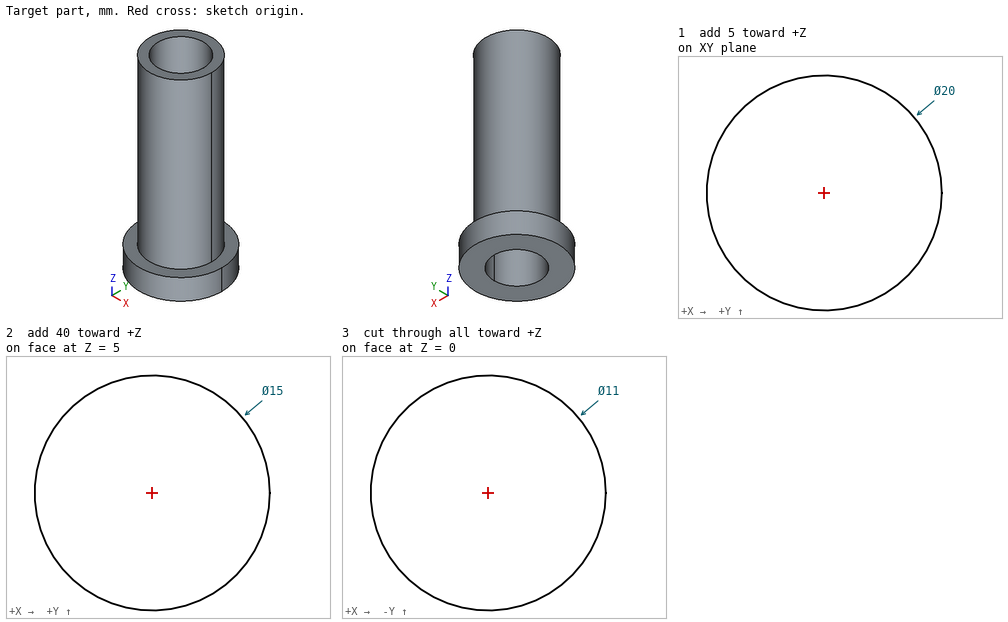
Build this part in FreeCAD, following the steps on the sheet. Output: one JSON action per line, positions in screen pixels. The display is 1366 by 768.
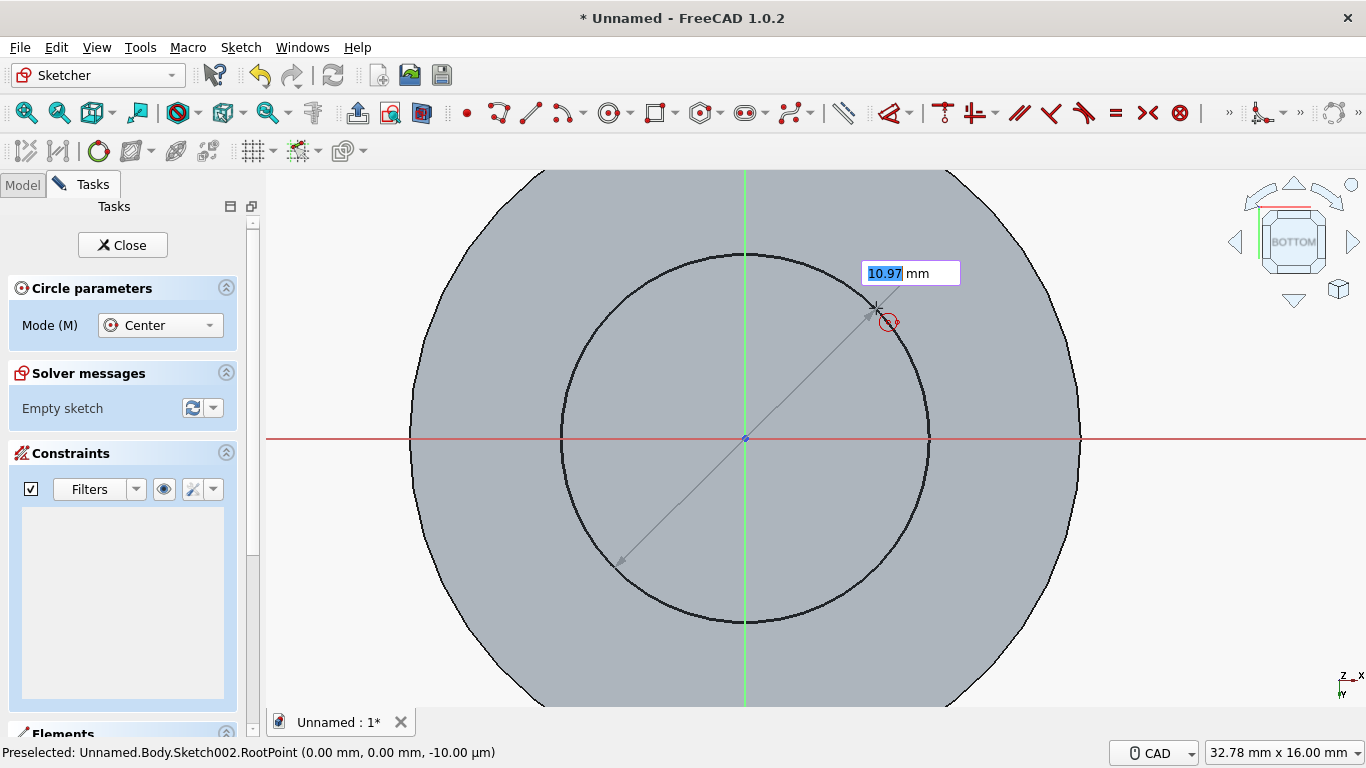
{"action": "type", "text": "11"}
{"action": "key", "text": "Return"}
{"action": "key", "text": "Escape"}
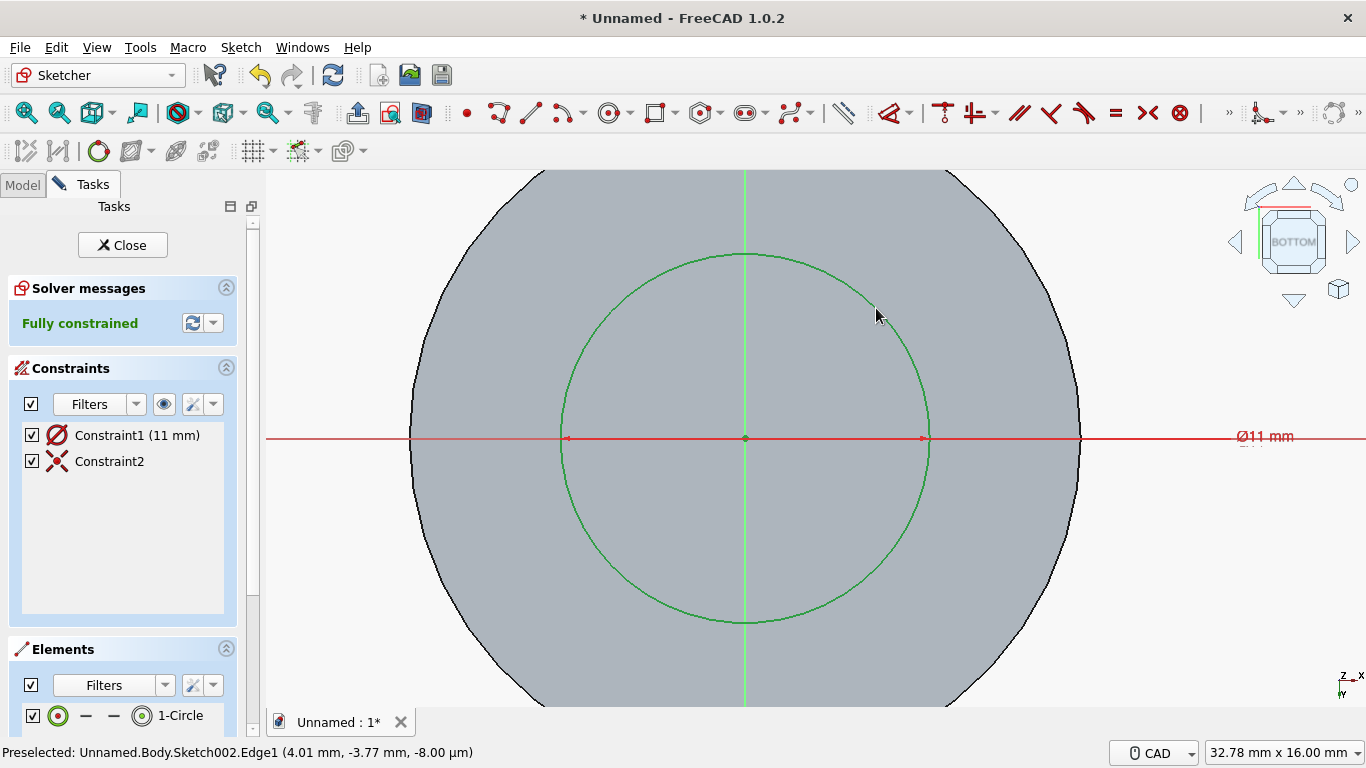
{"action": "left_click", "coordinate": [123, 245]}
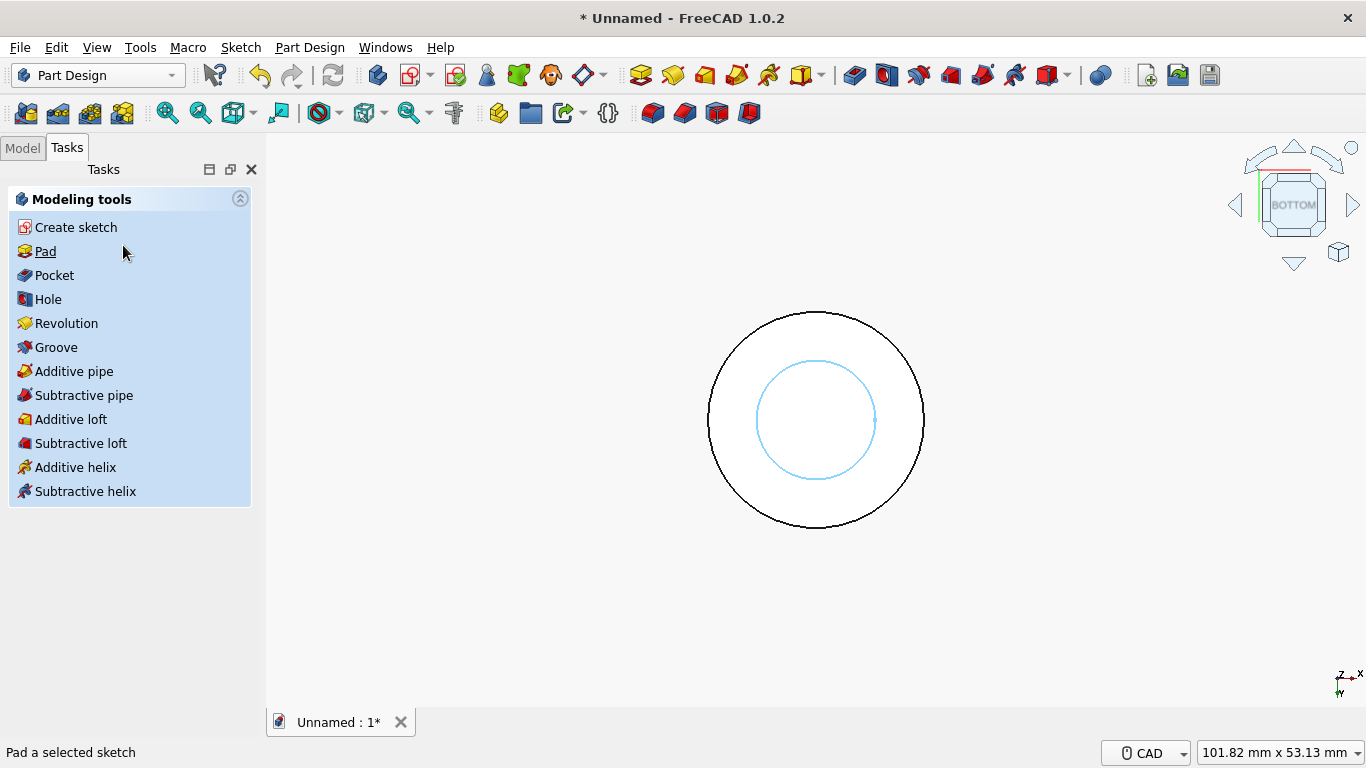
{"action": "left_click", "coordinate": [856, 76]}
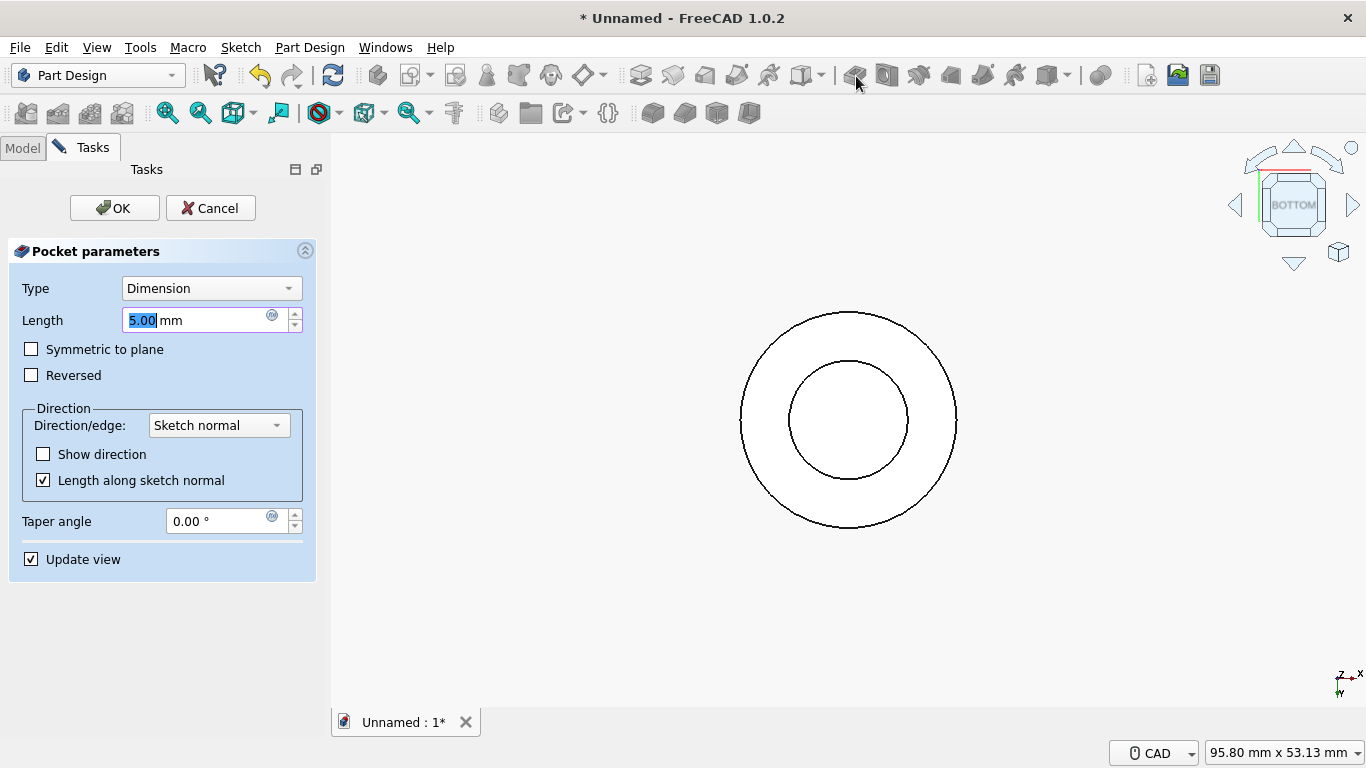
{"action": "left_click", "coordinate": [212, 288]}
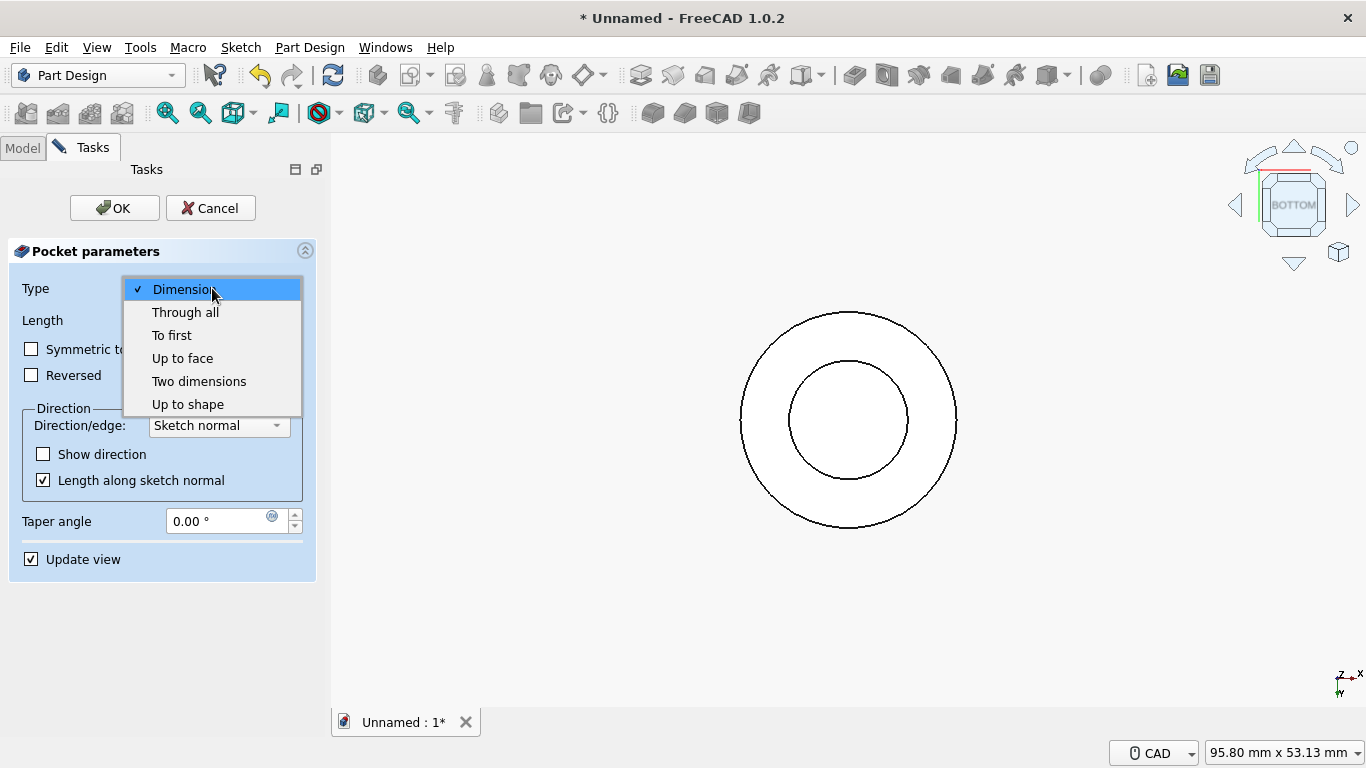
{"action": "left_click", "coordinate": [212, 312]}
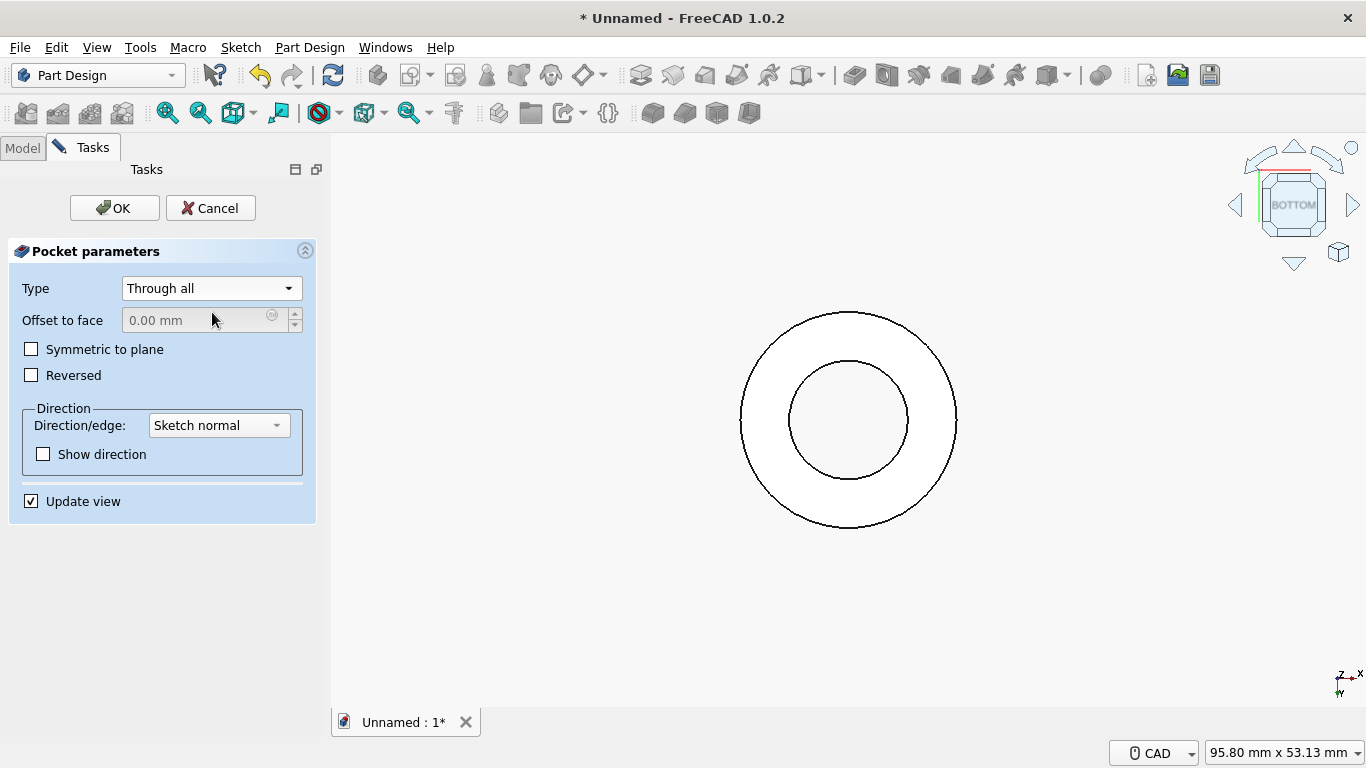
{"action": "left_click", "coordinate": [115, 208]}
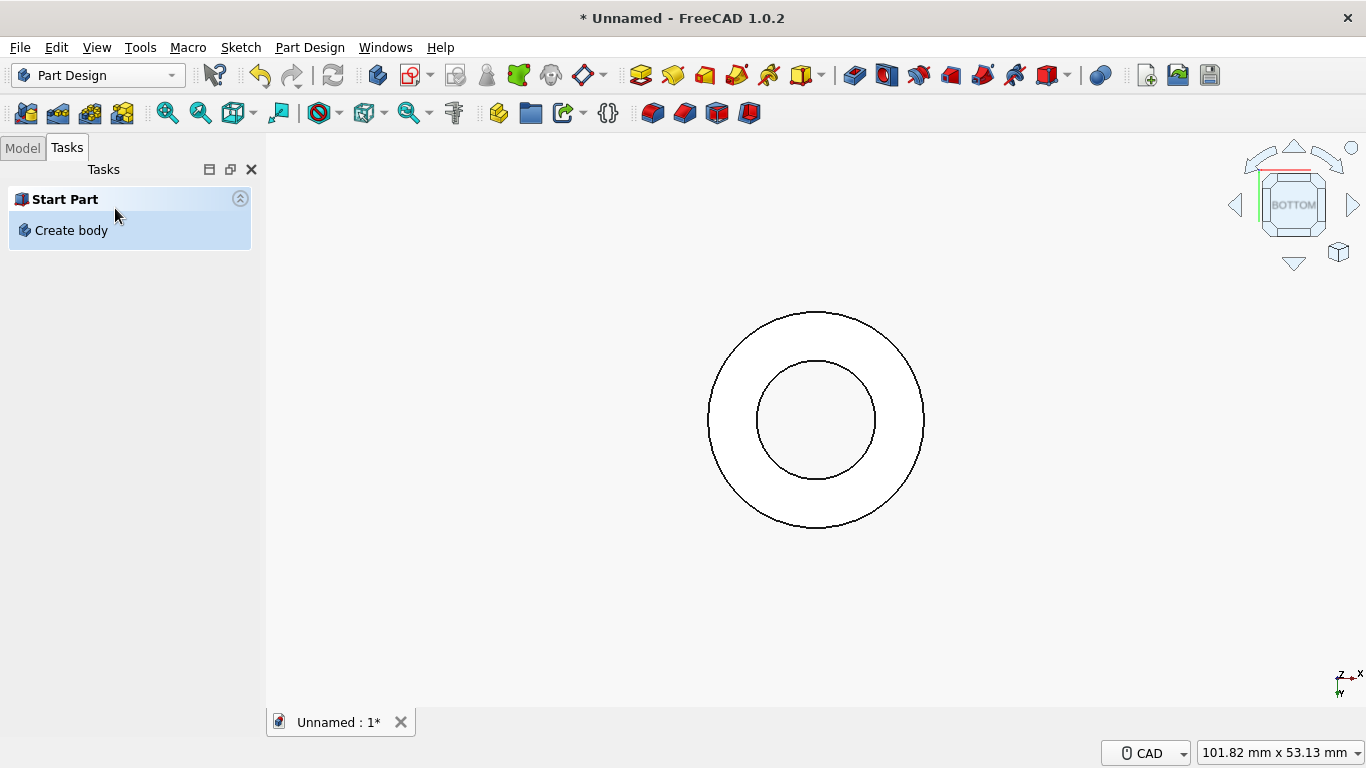
{"action": "key", "text": "0"}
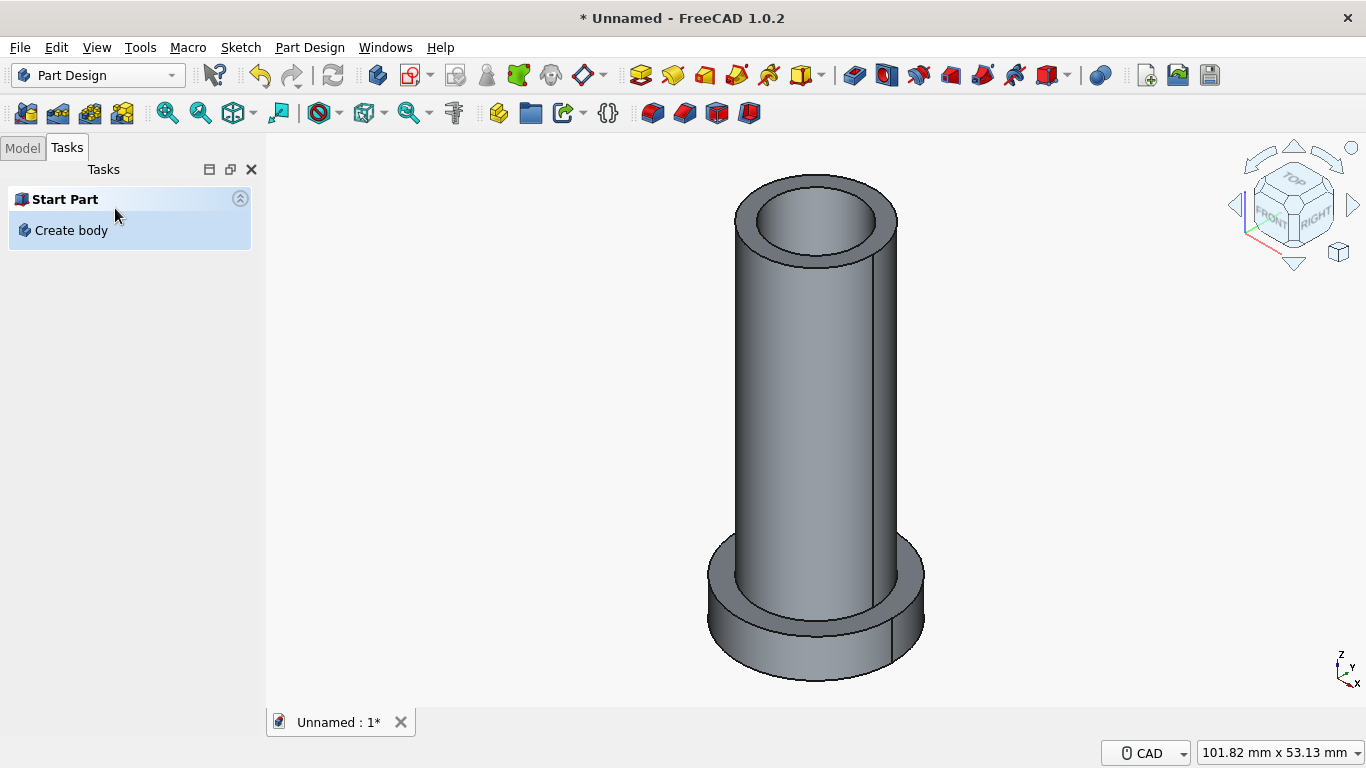
{"action": "left_click", "coordinate": [168, 114]}